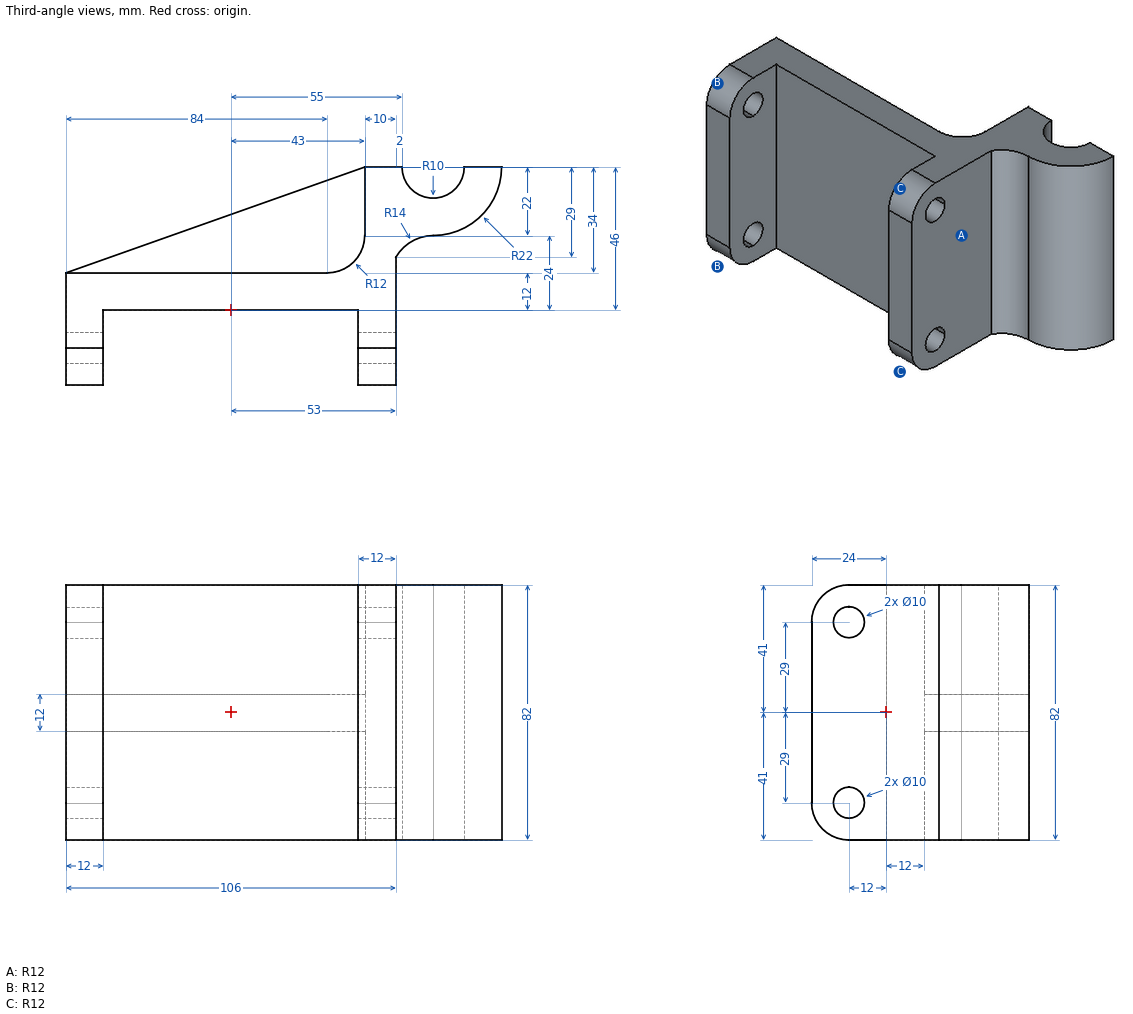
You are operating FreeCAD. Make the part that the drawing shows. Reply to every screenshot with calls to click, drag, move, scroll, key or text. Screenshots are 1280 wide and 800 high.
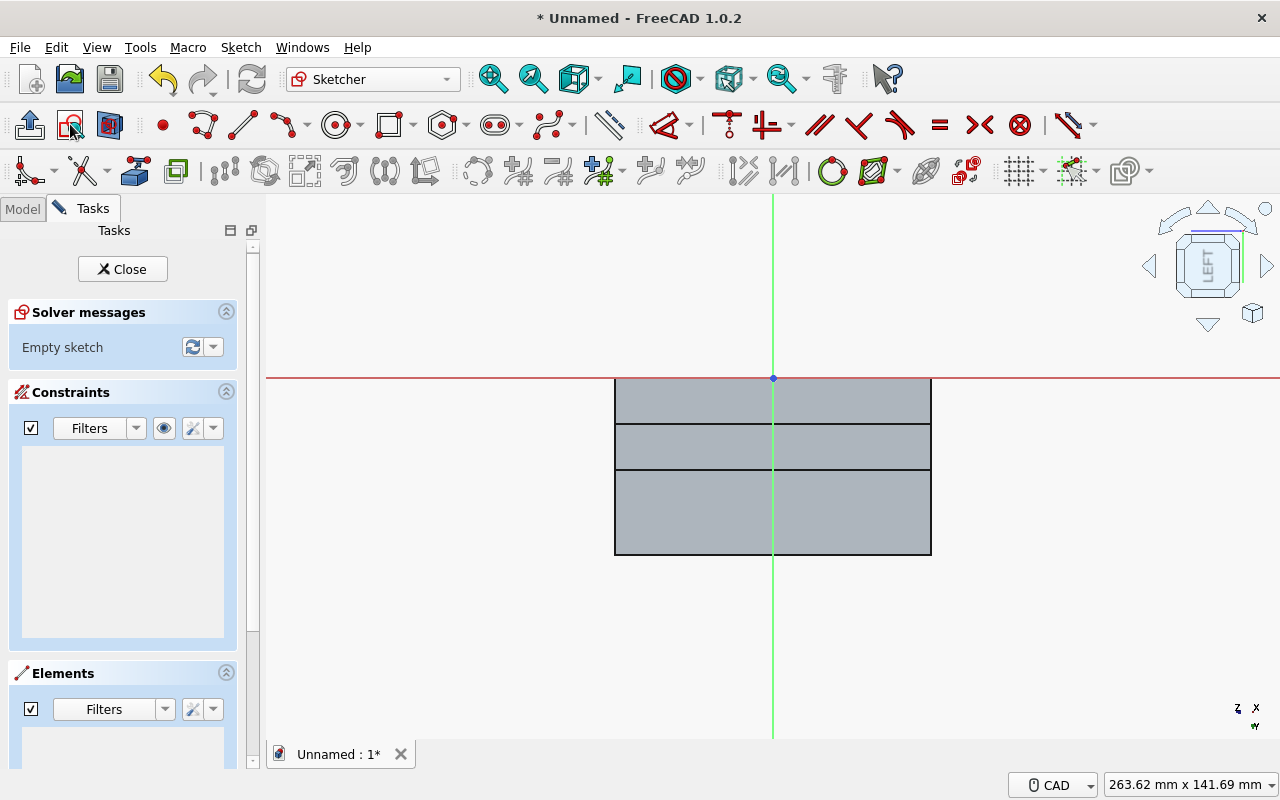
scroll(856, 222, up, 3)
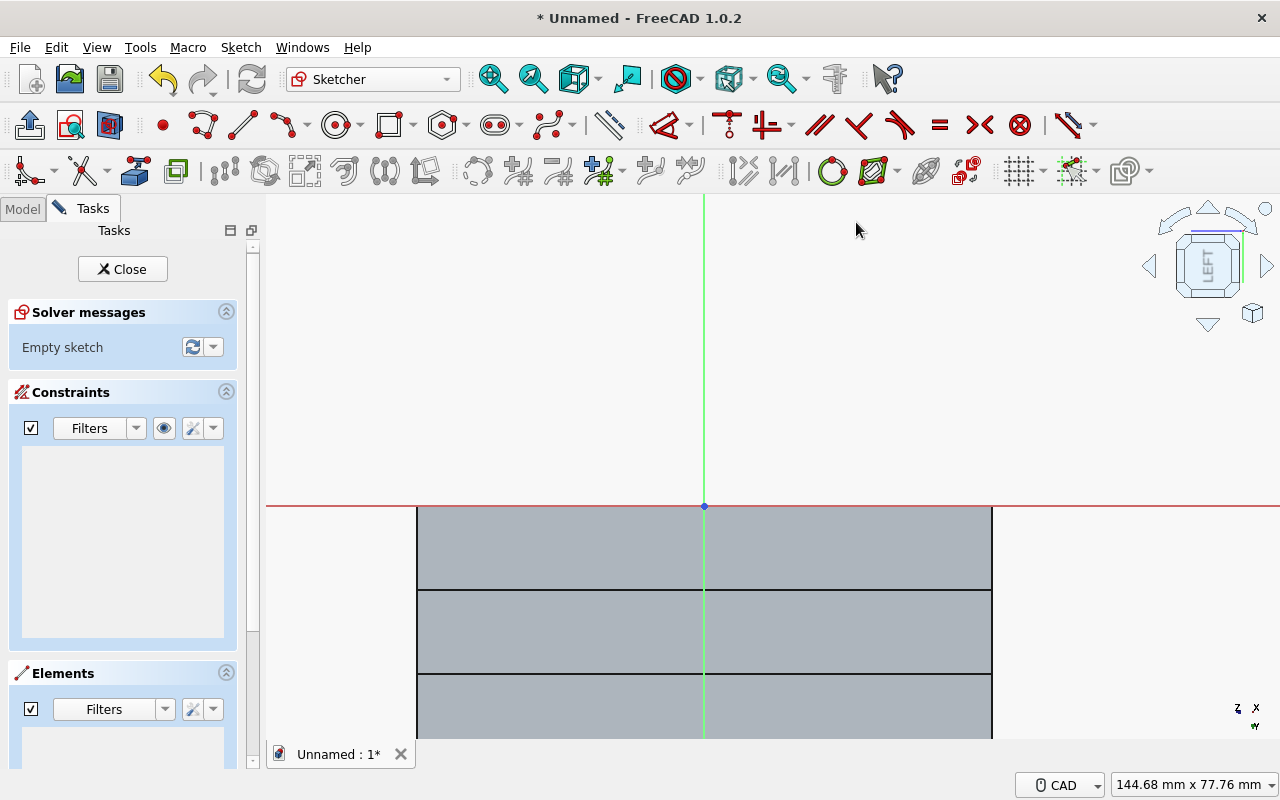
key(g)
key(r)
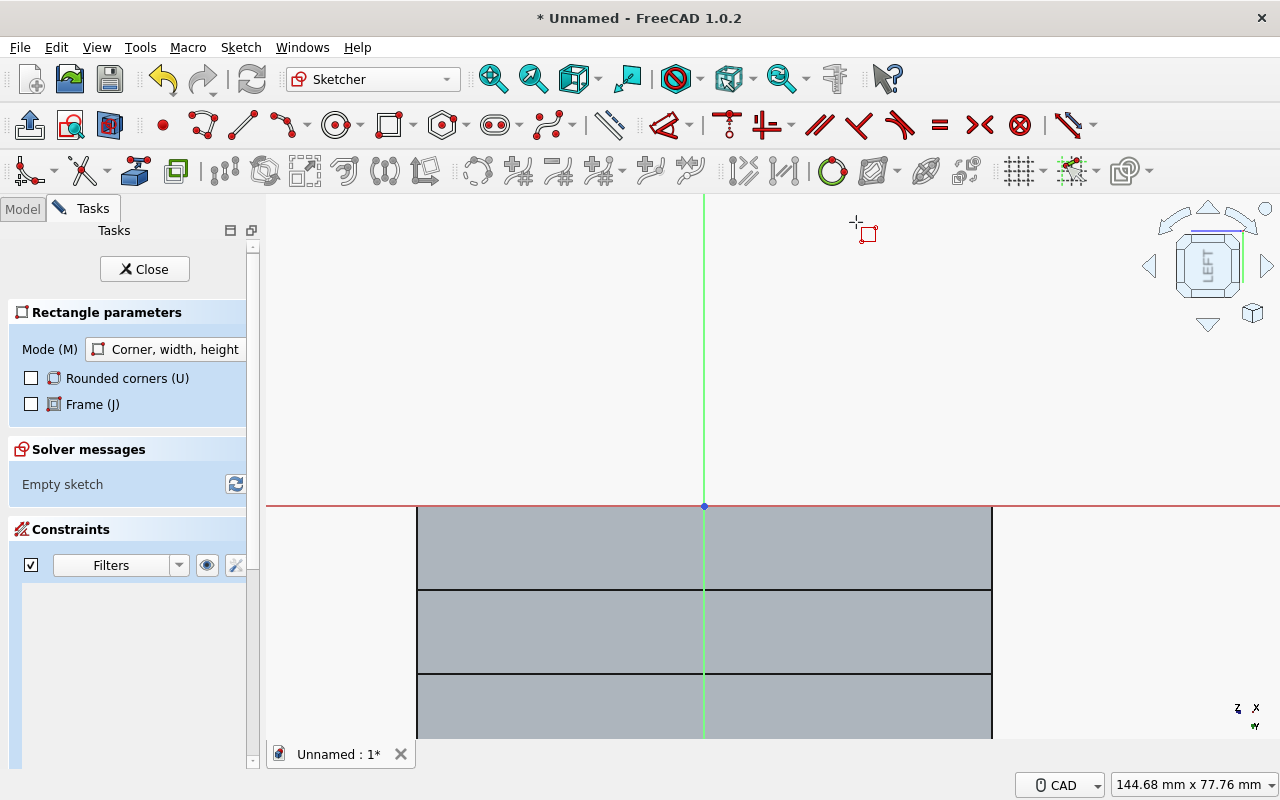
click(417, 338)
click(992, 506)
key(Escape)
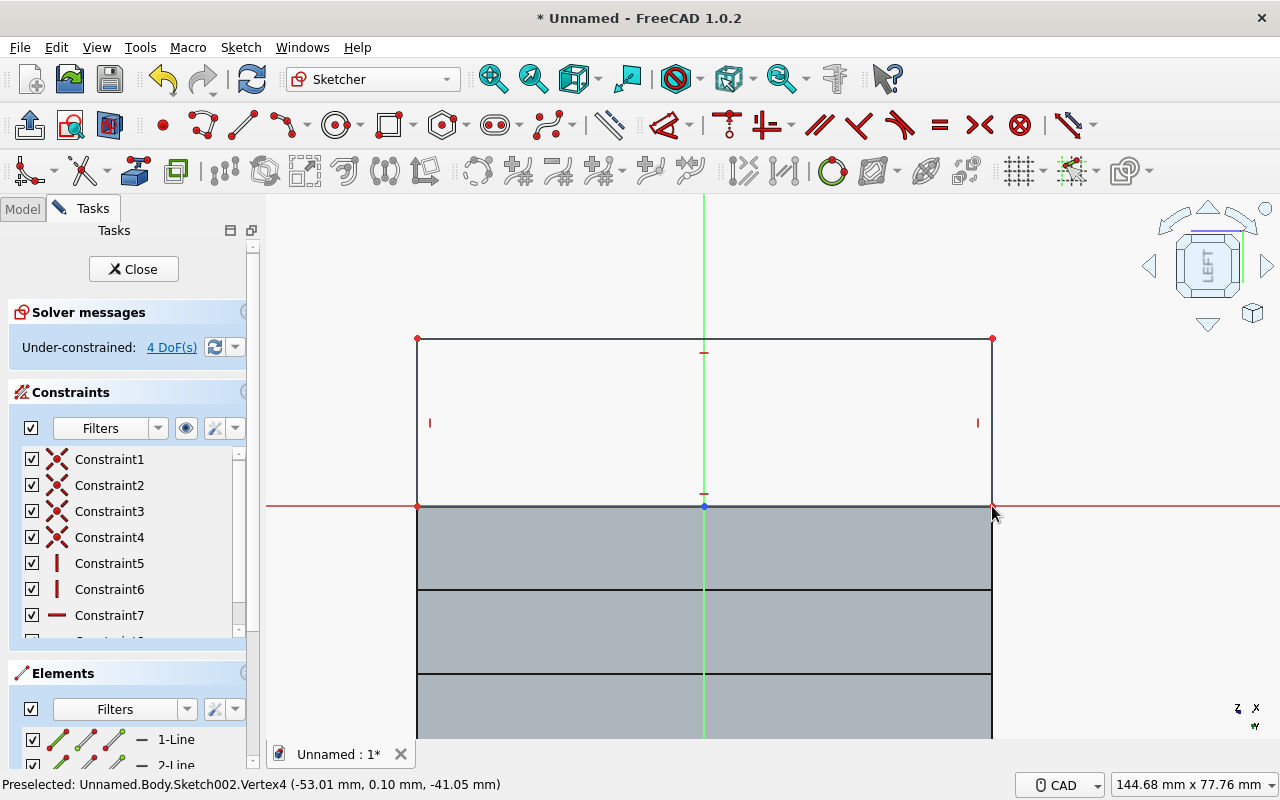
click(417, 507)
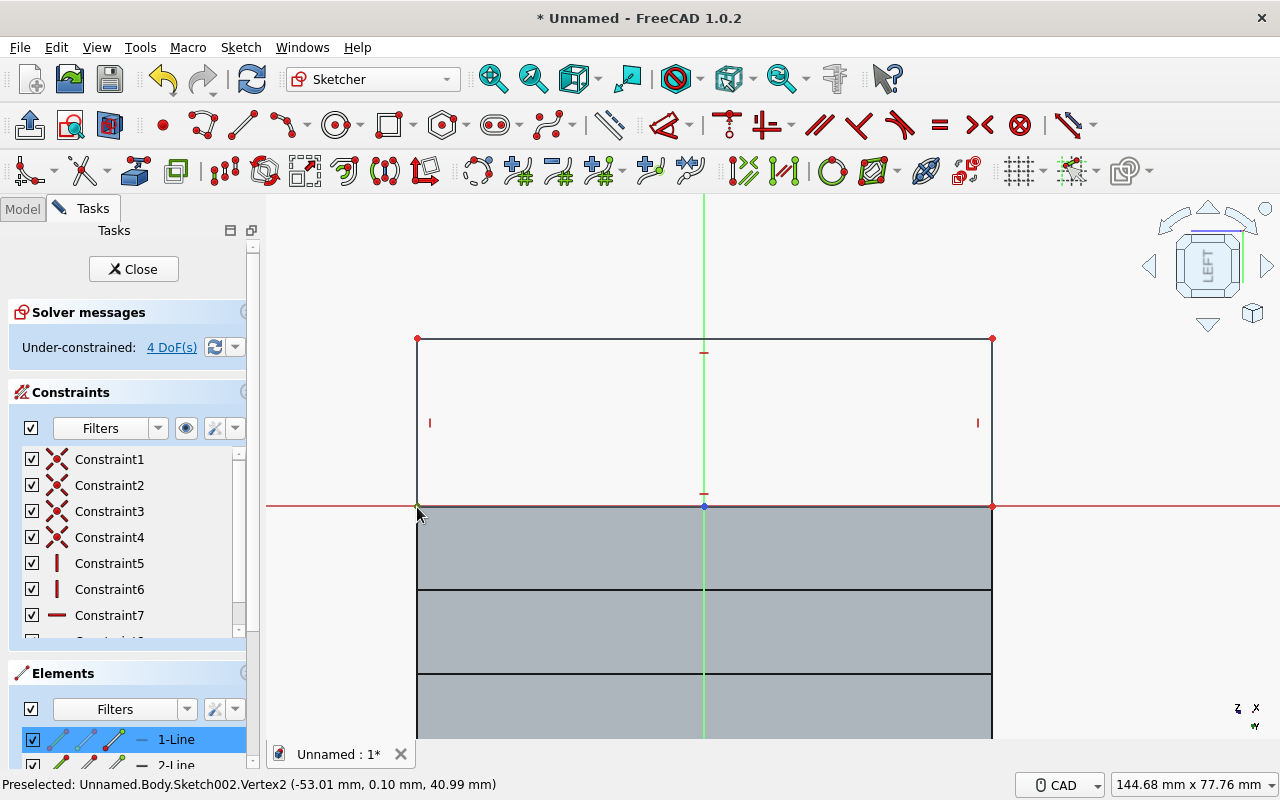
click(353, 506)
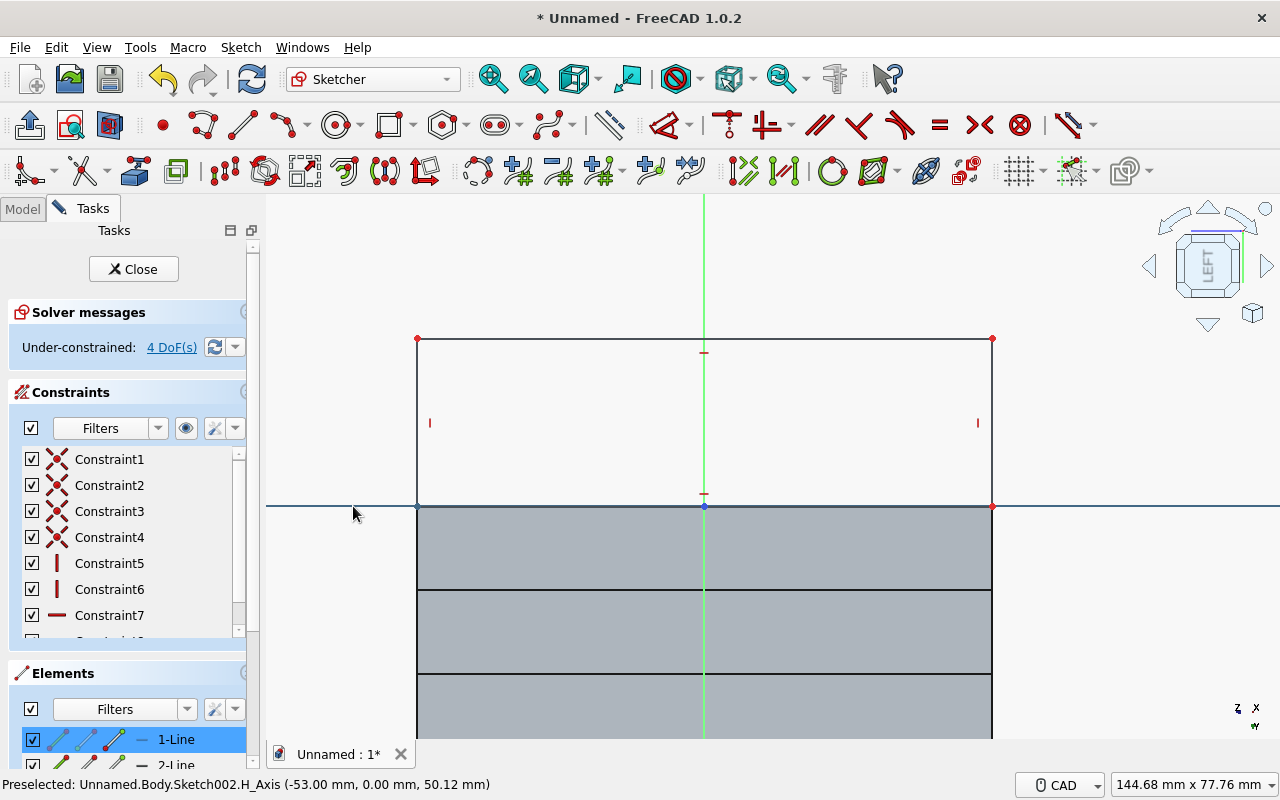
key(c)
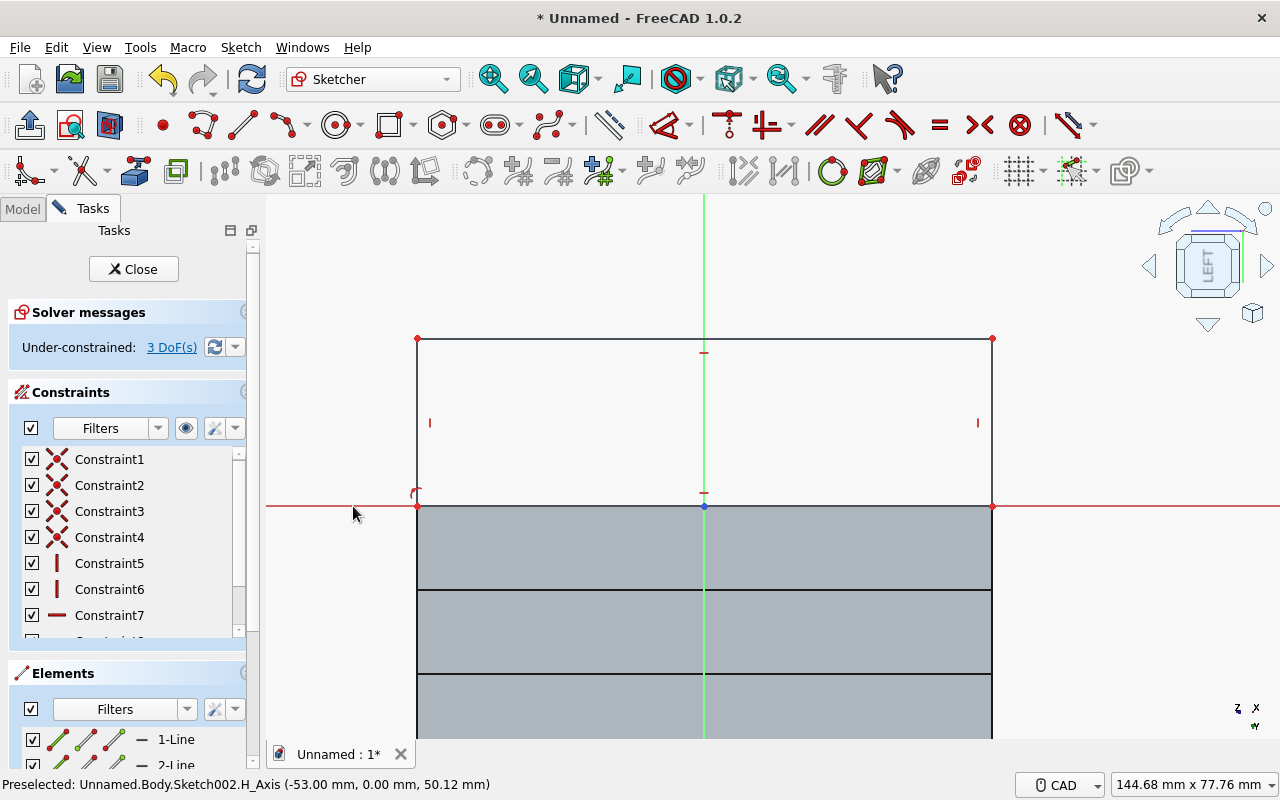
click(664, 126)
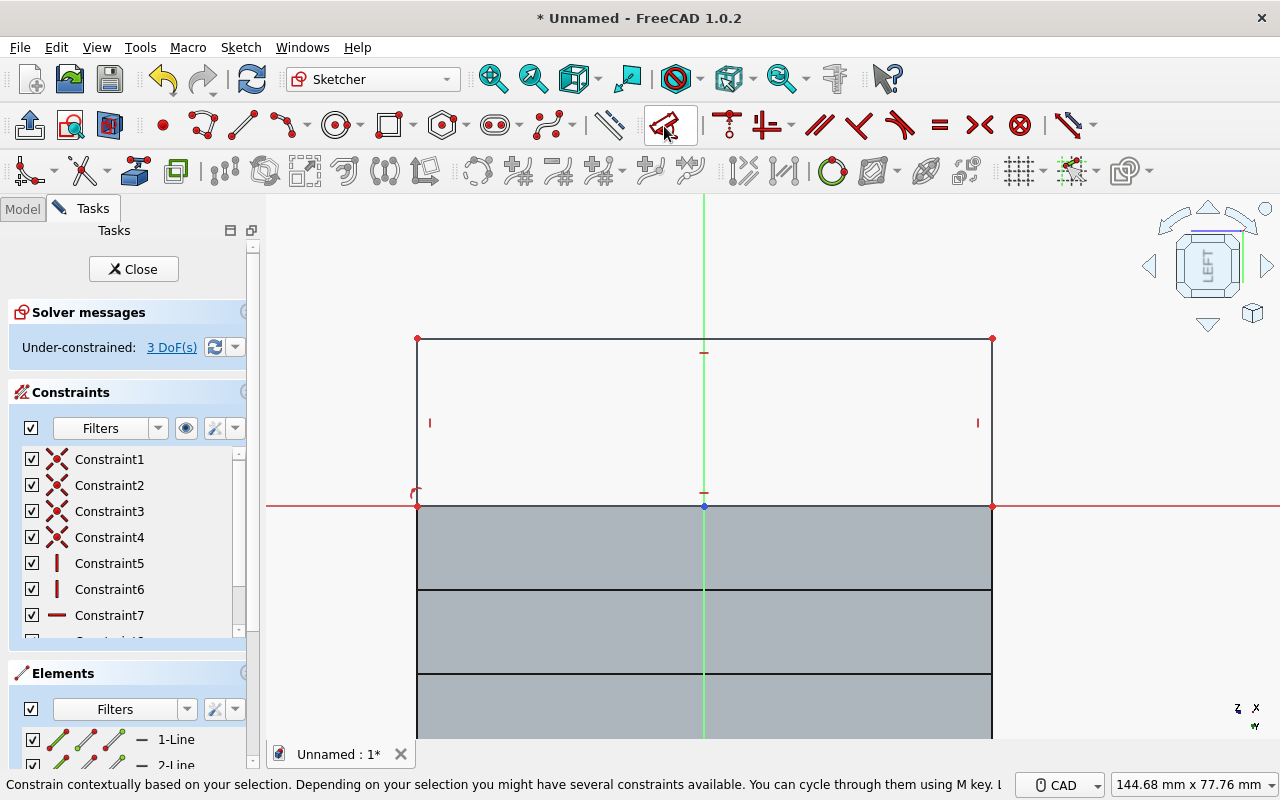
click(417, 389)
click(383, 423)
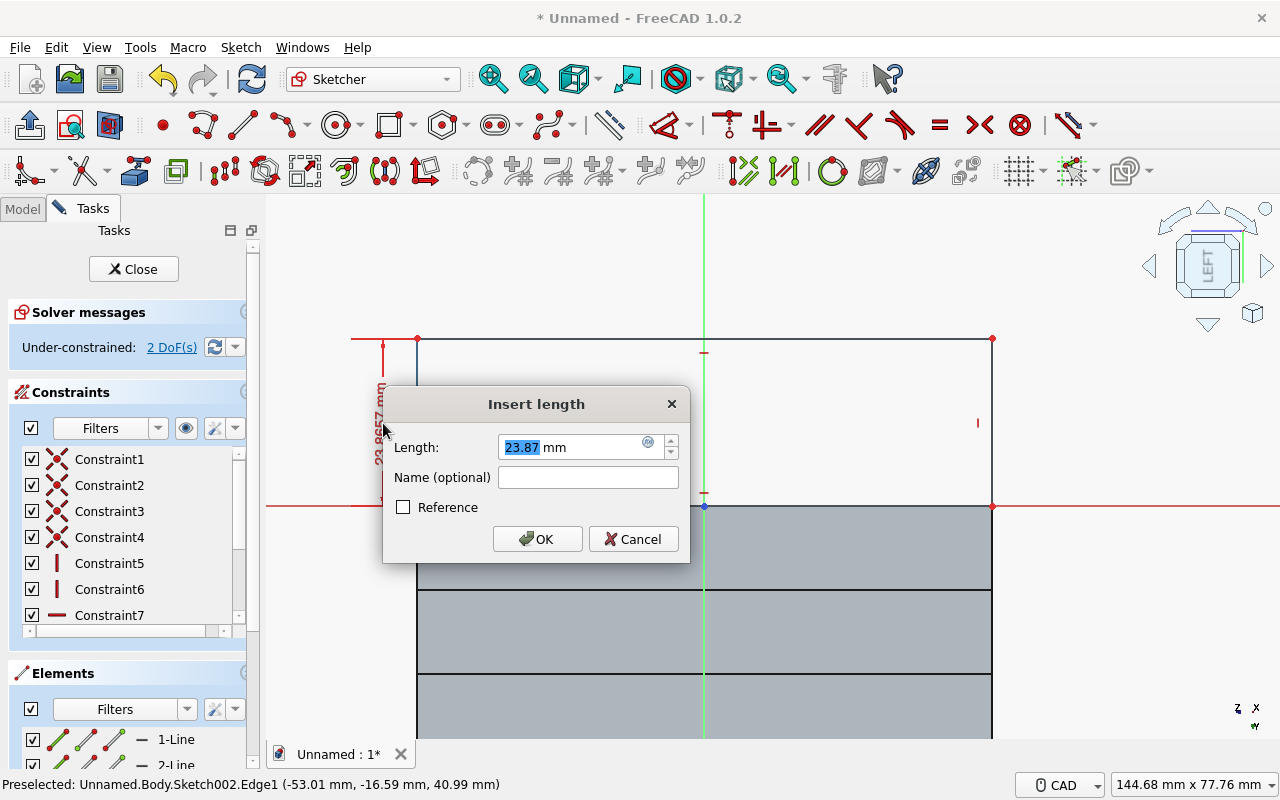
text(24)
key(Return)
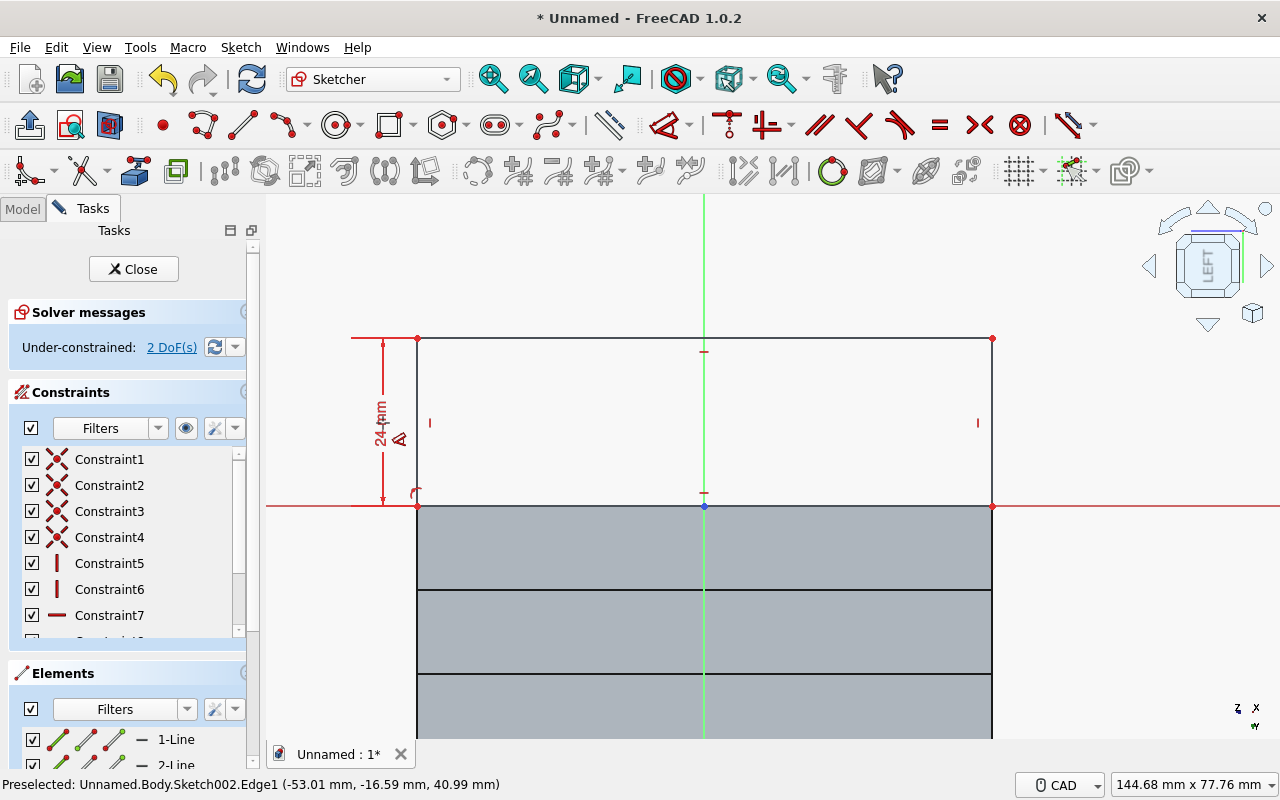
click(590, 506)
click(572, 540)